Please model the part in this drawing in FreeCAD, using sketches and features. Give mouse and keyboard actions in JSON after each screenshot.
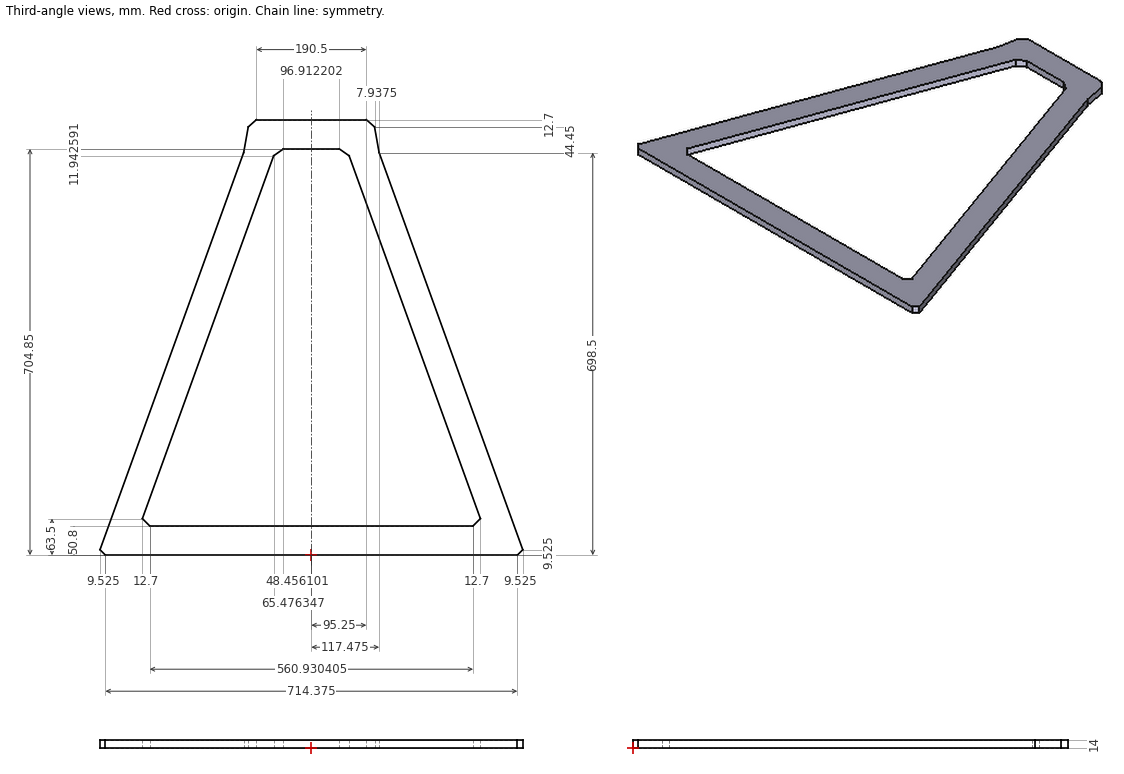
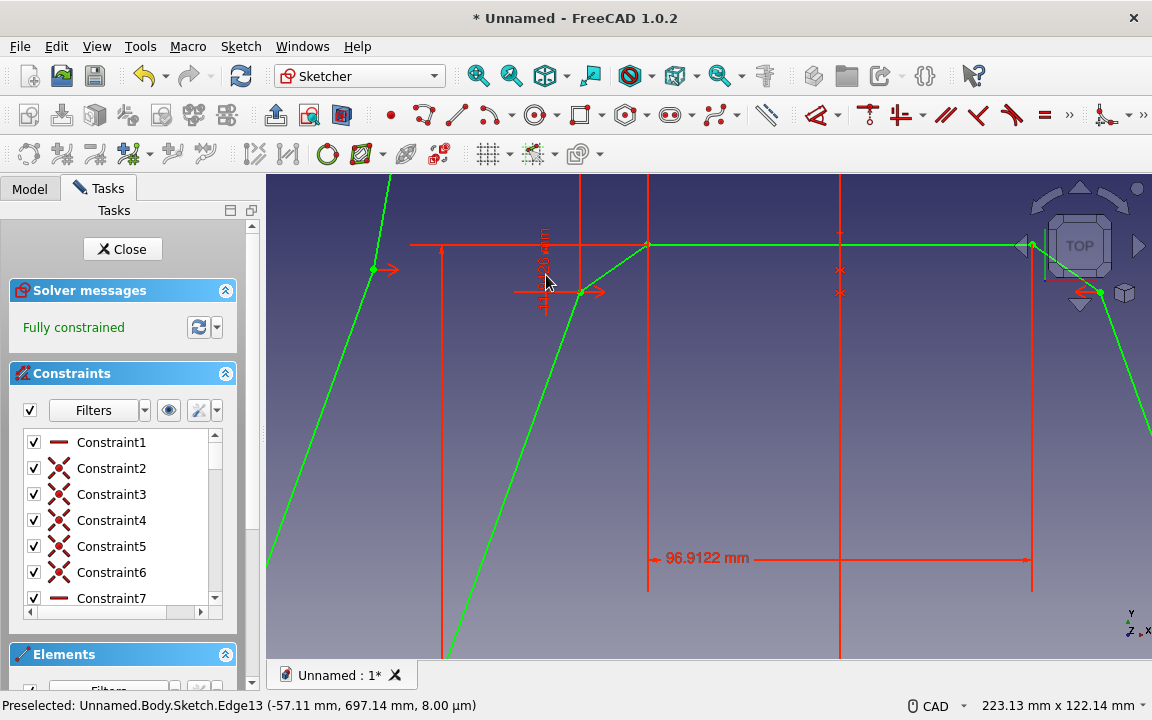
{"action": "left_click", "coordinate": [123, 249]}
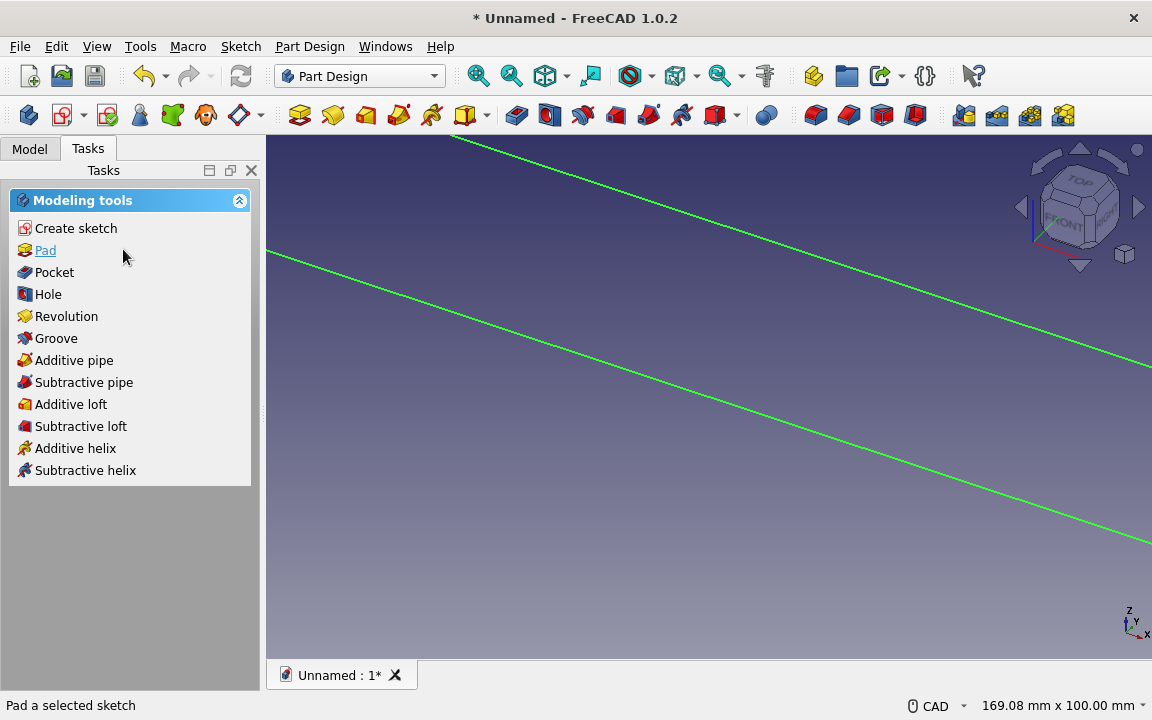
{"action": "left_click", "coordinate": [300, 116]}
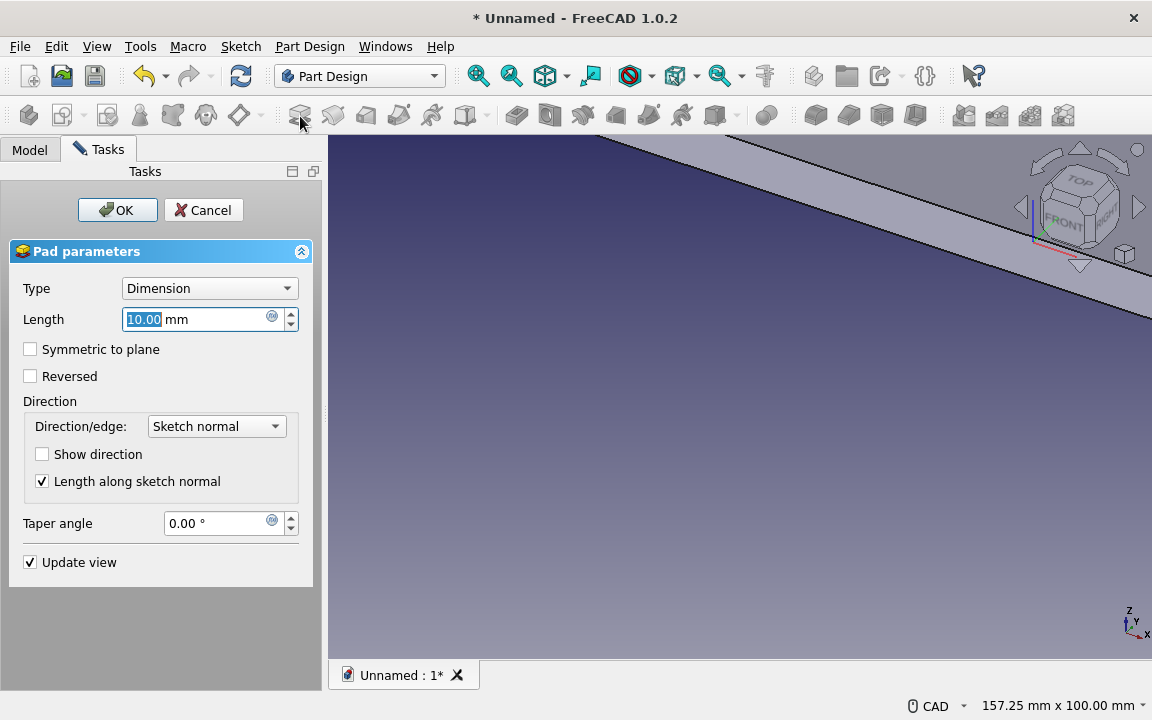
{"action": "type", "text": "14"}
{"action": "key", "text": "Tab"}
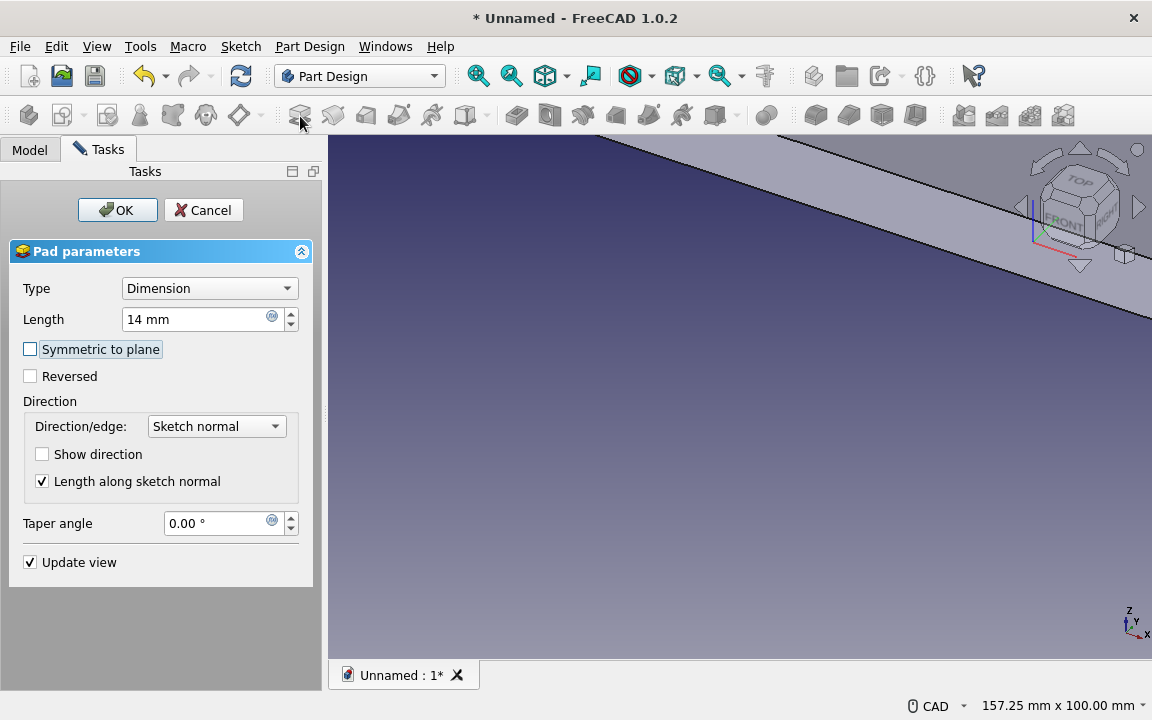
{"action": "left_click", "coordinate": [118, 210]}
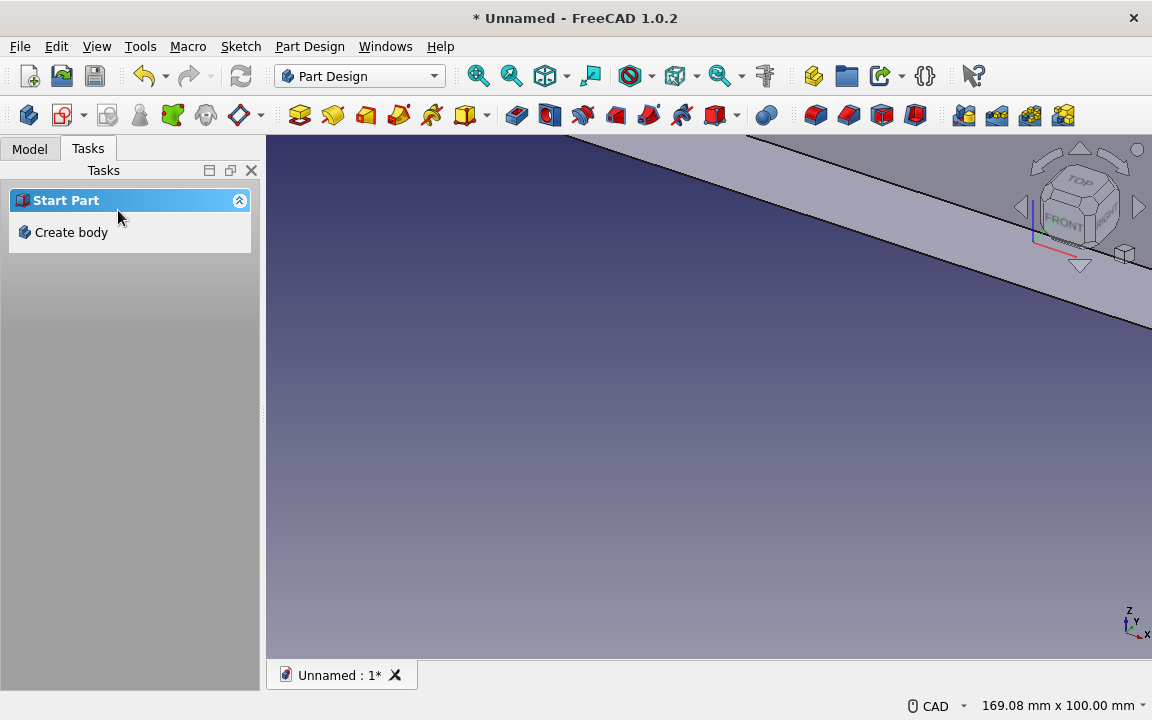
{"action": "key", "text": "0"}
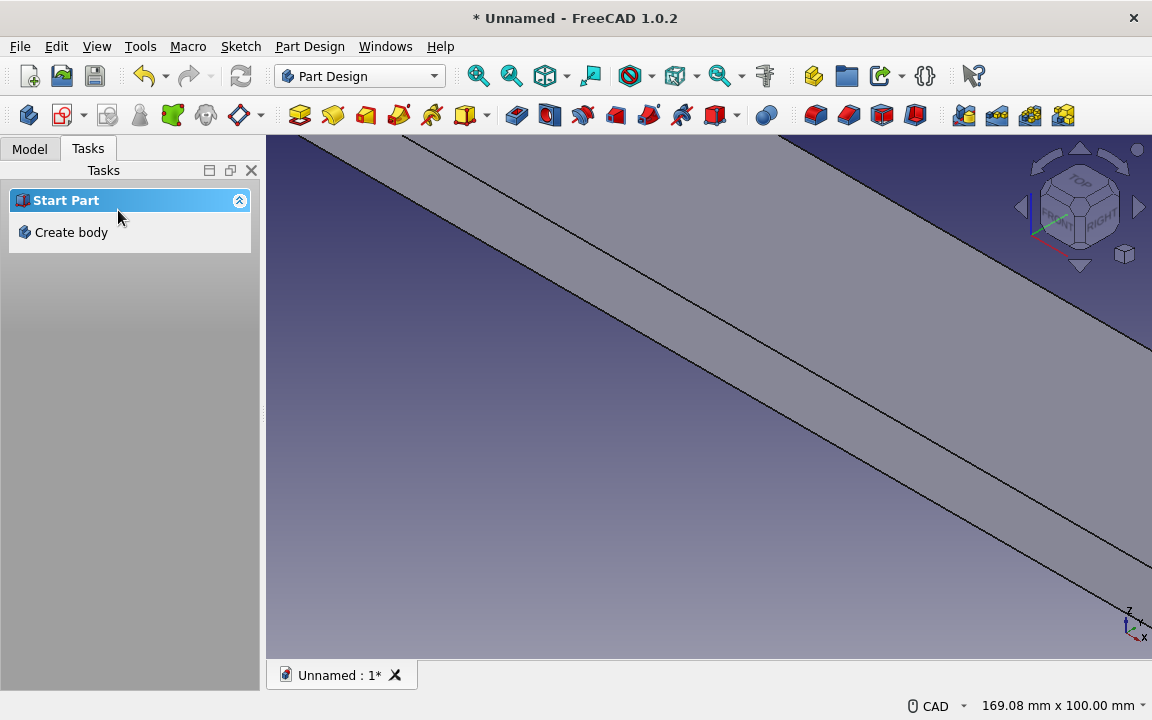
{"action": "left_click", "coordinate": [479, 76]}